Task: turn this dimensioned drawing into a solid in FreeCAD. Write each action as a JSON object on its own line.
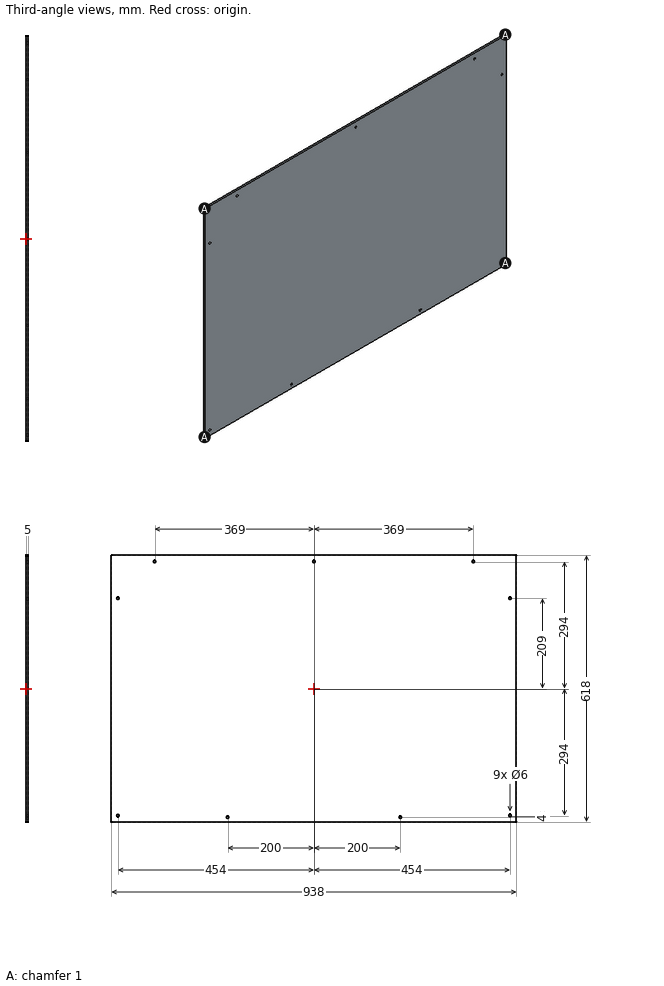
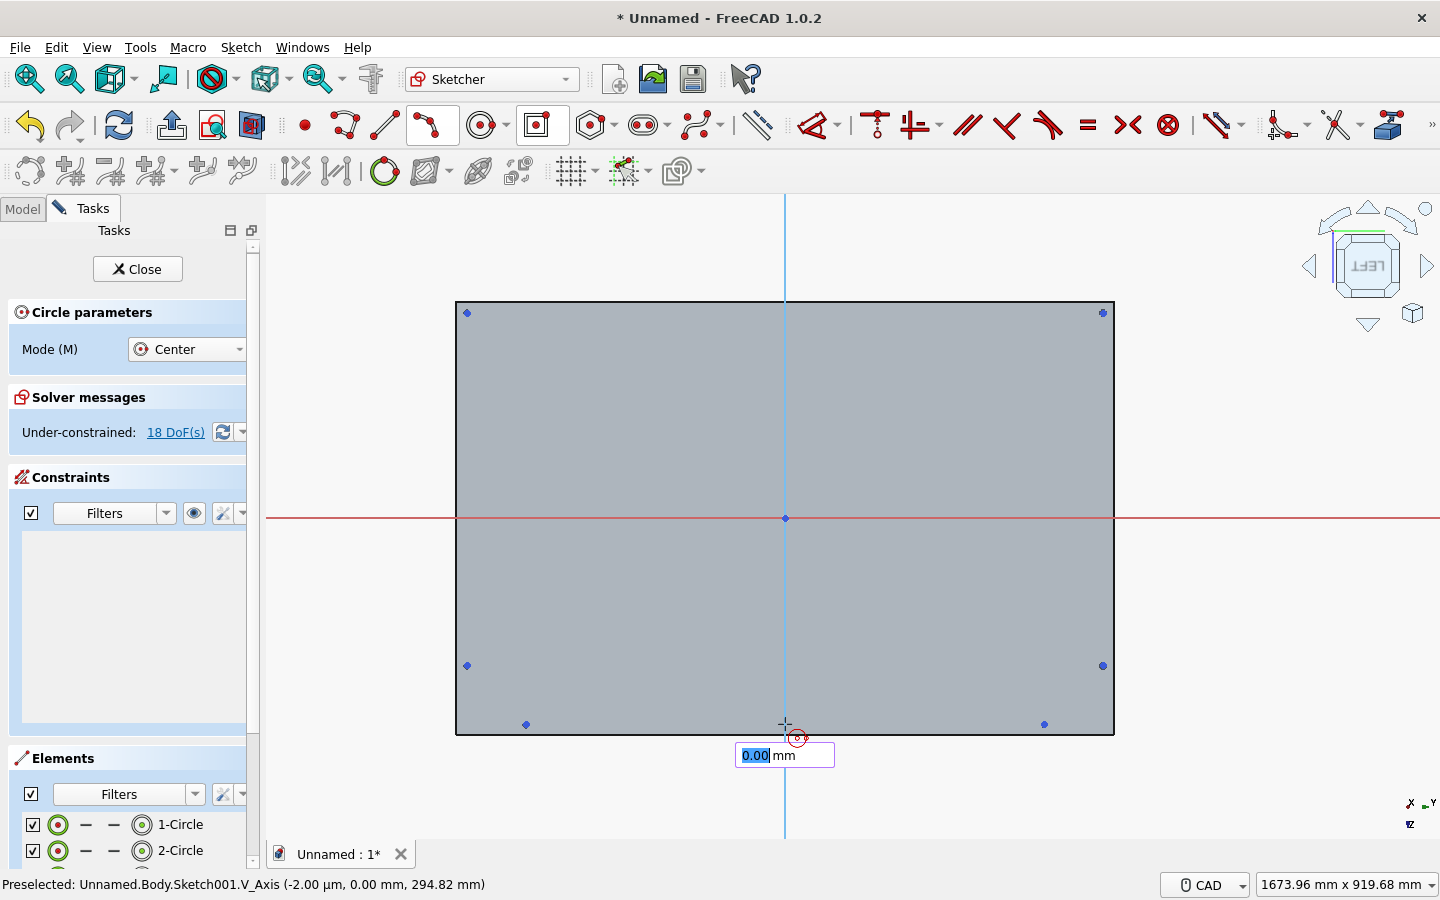
{"action": "scroll", "coordinate": [787, 724], "scroll_direction": "up", "scroll_amount": 11}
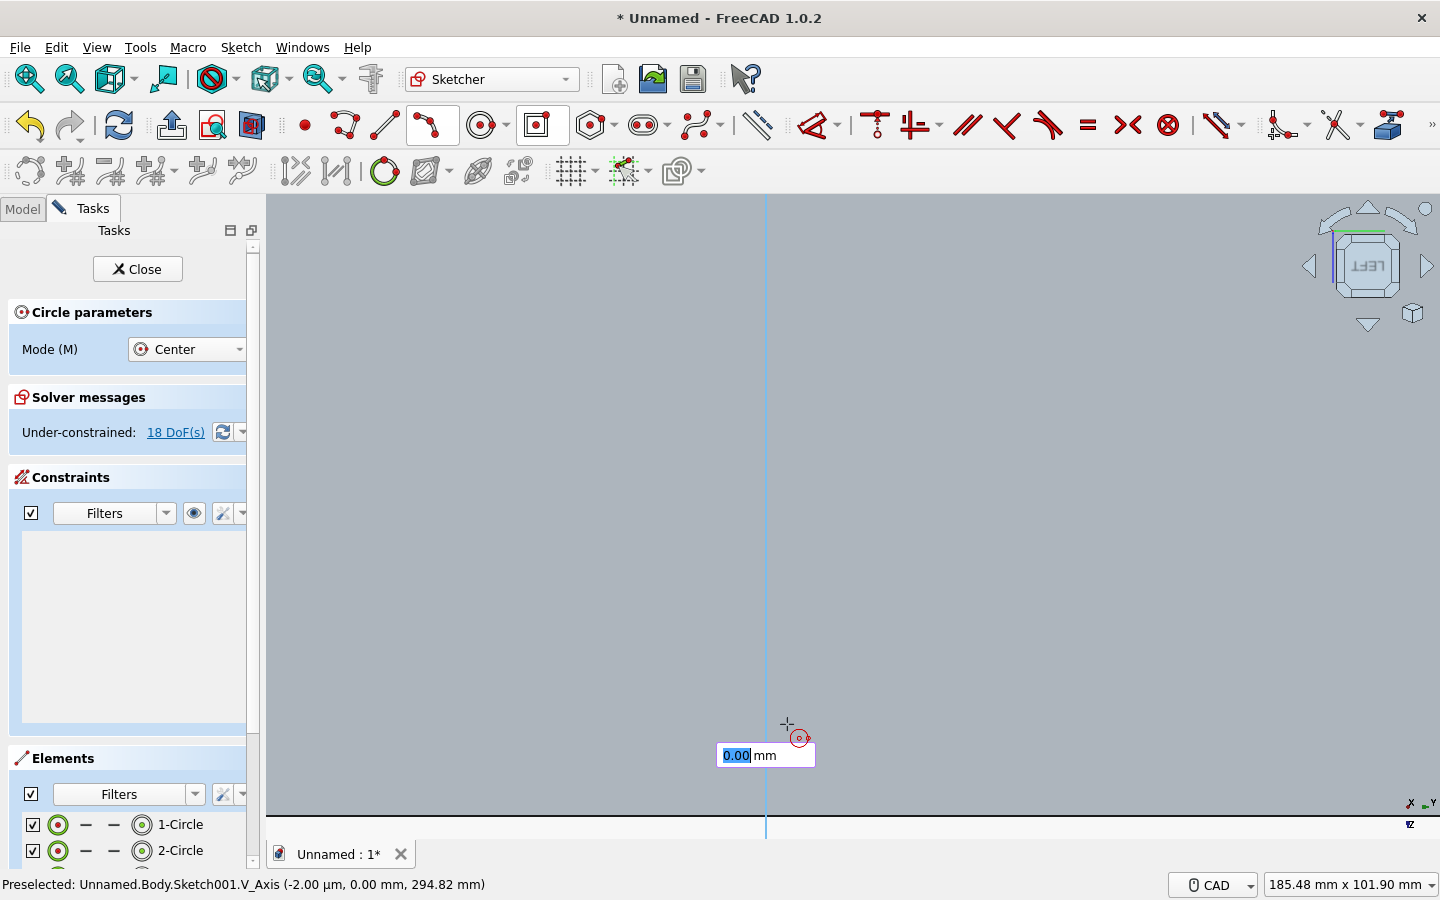
{"action": "left_click", "coordinate": [784, 715]}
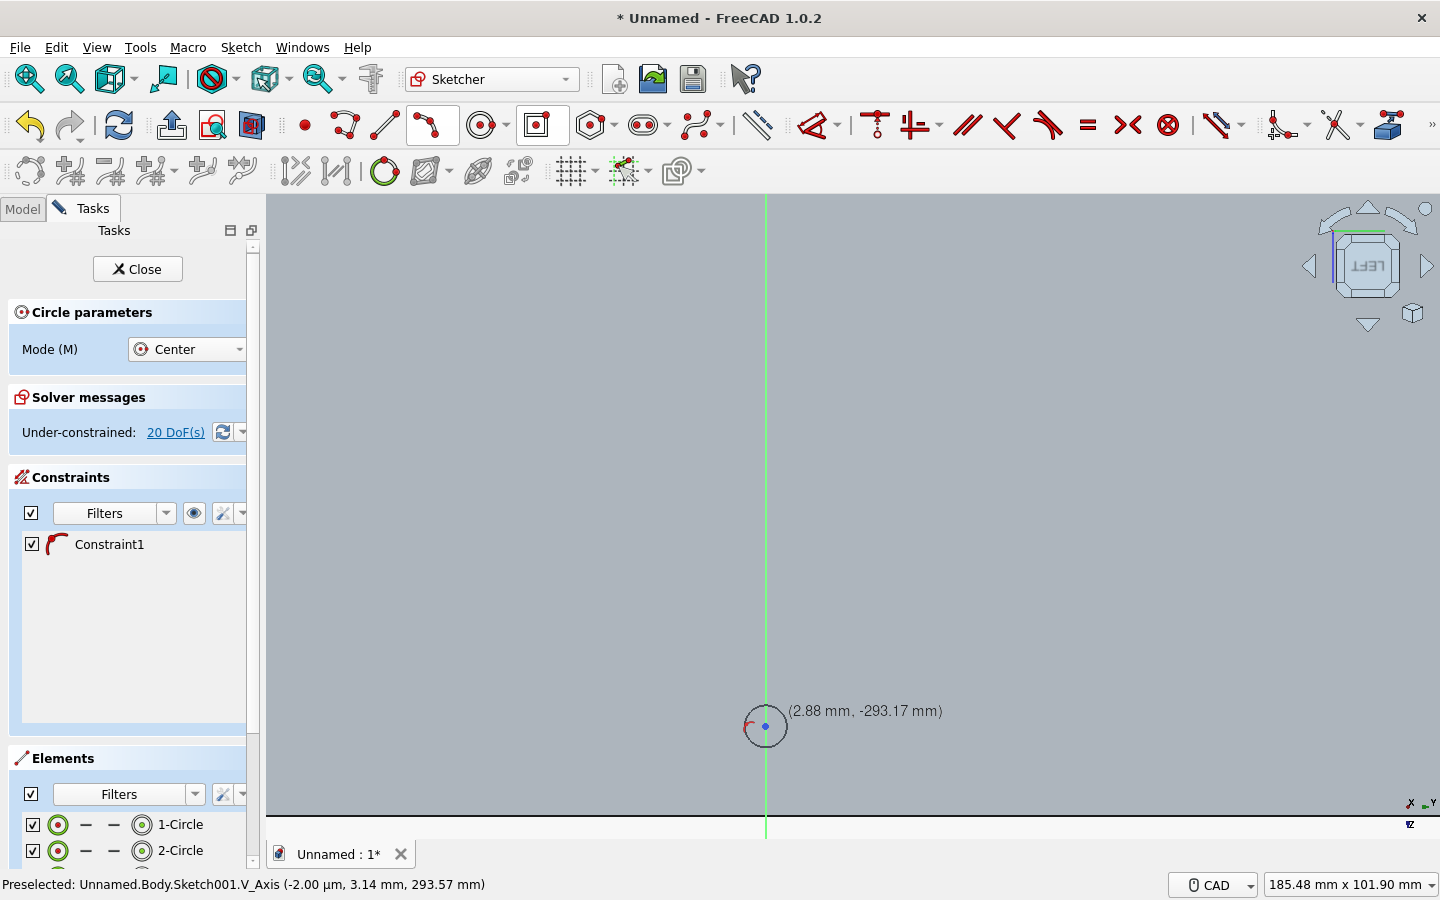
{"action": "scroll", "coordinate": [787, 724], "scroll_direction": "down", "scroll_amount": 11}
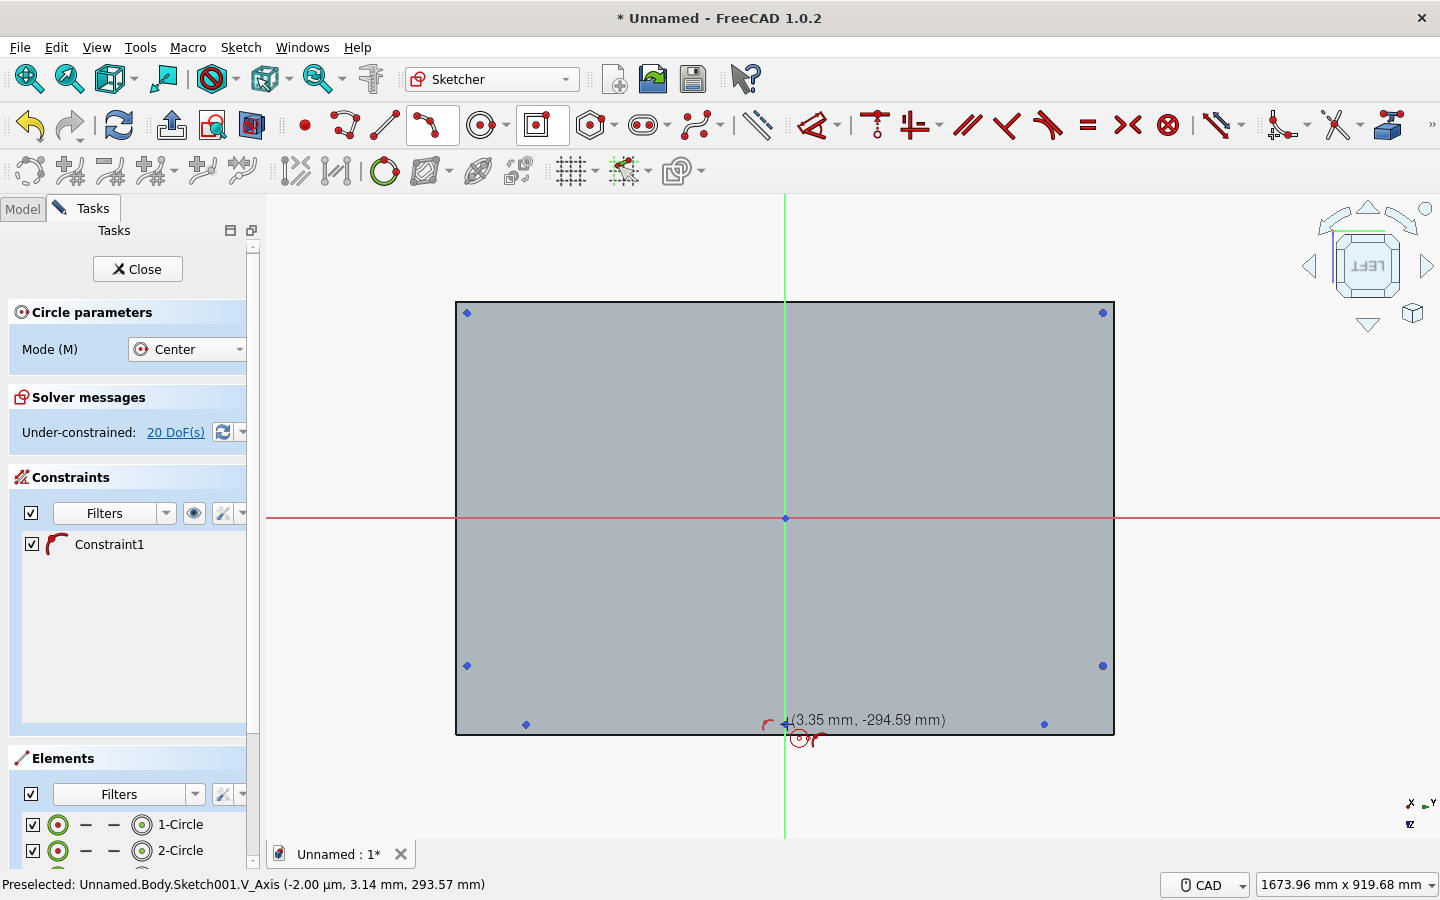
{"action": "scroll", "coordinate": [925, 309], "scroll_direction": "up", "scroll_amount": 12}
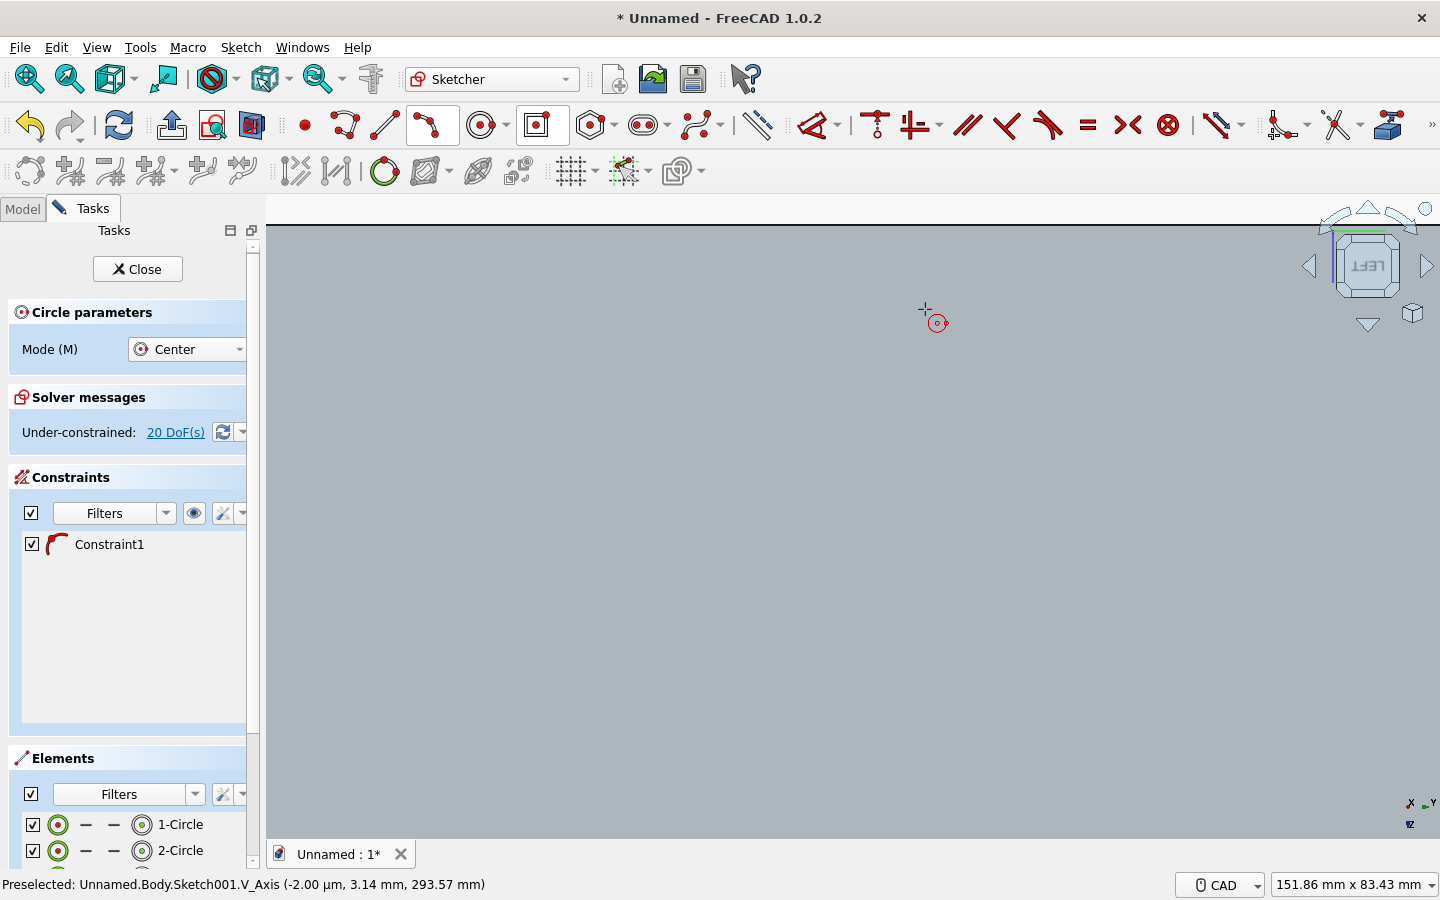
{"action": "scroll", "coordinate": [925, 309], "scroll_direction": "down", "scroll_amount": 12}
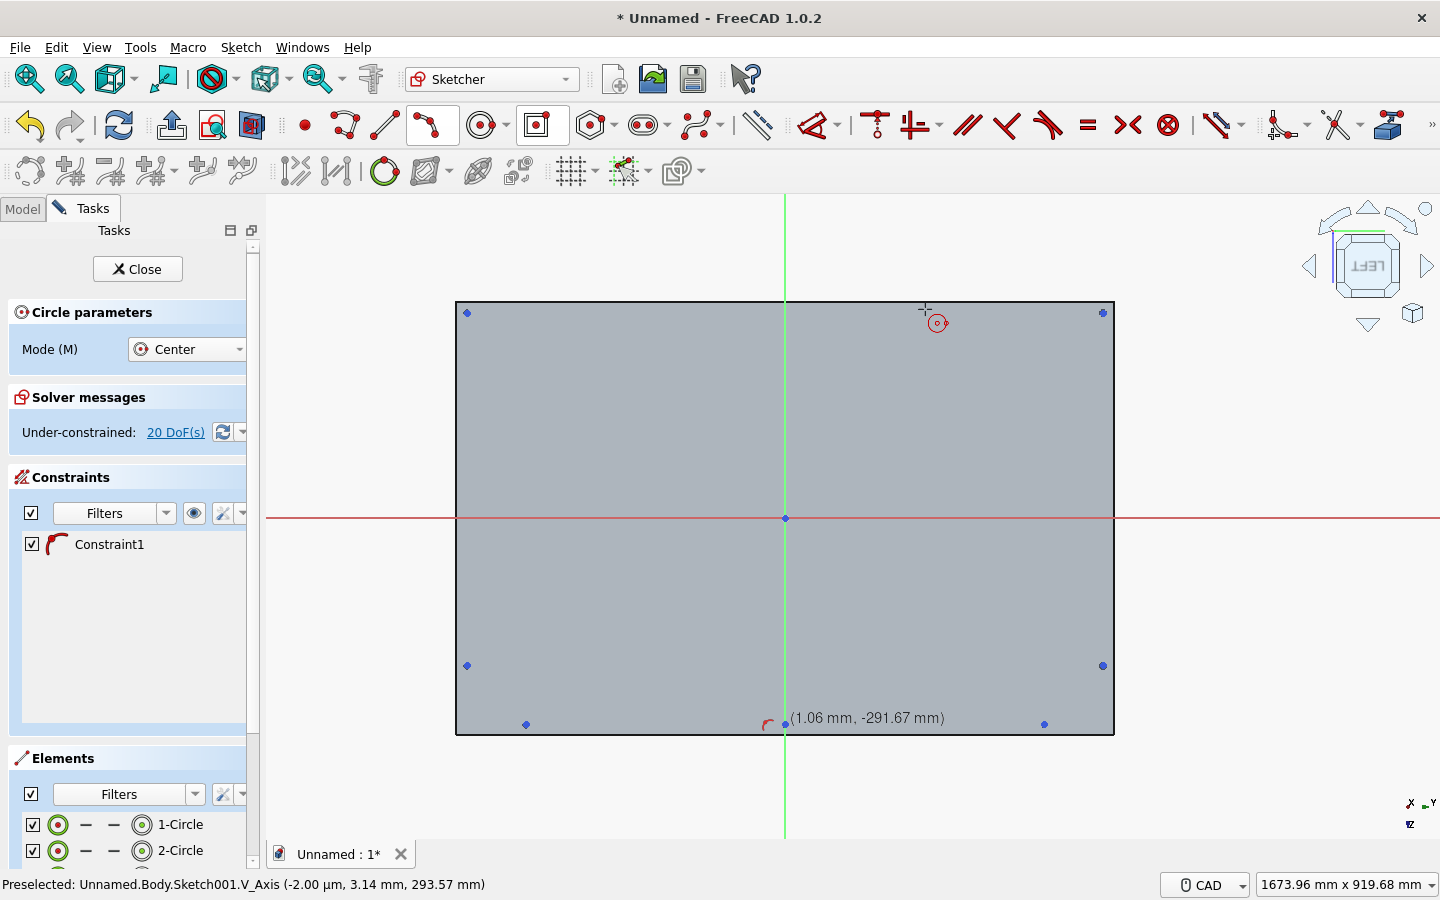
{"action": "left_click", "coordinate": [925, 309]}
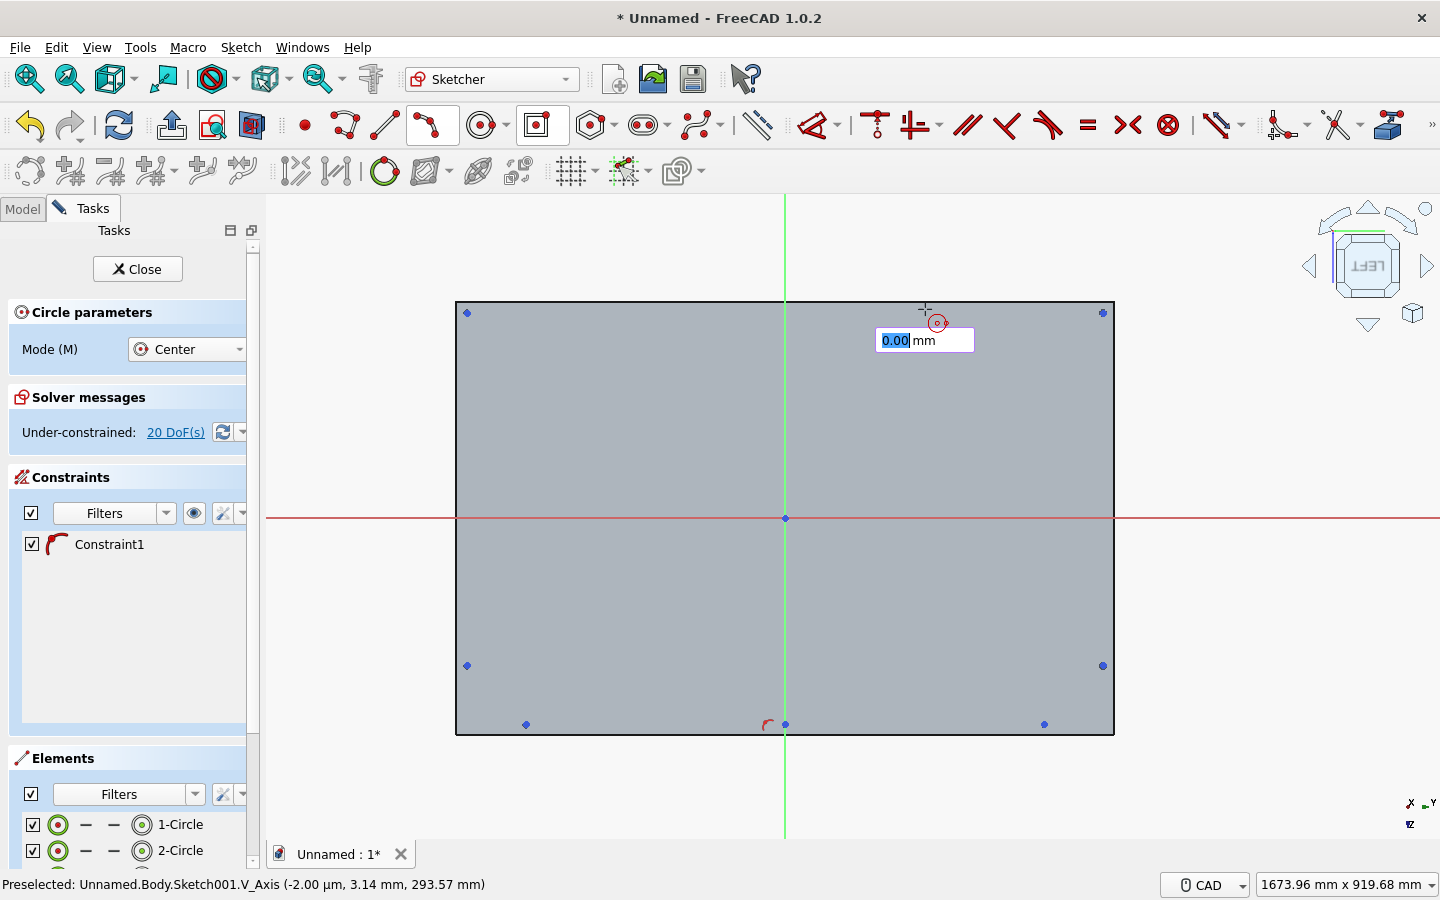
{"action": "scroll", "coordinate": [927, 308], "scroll_direction": "up", "scroll_amount": 11}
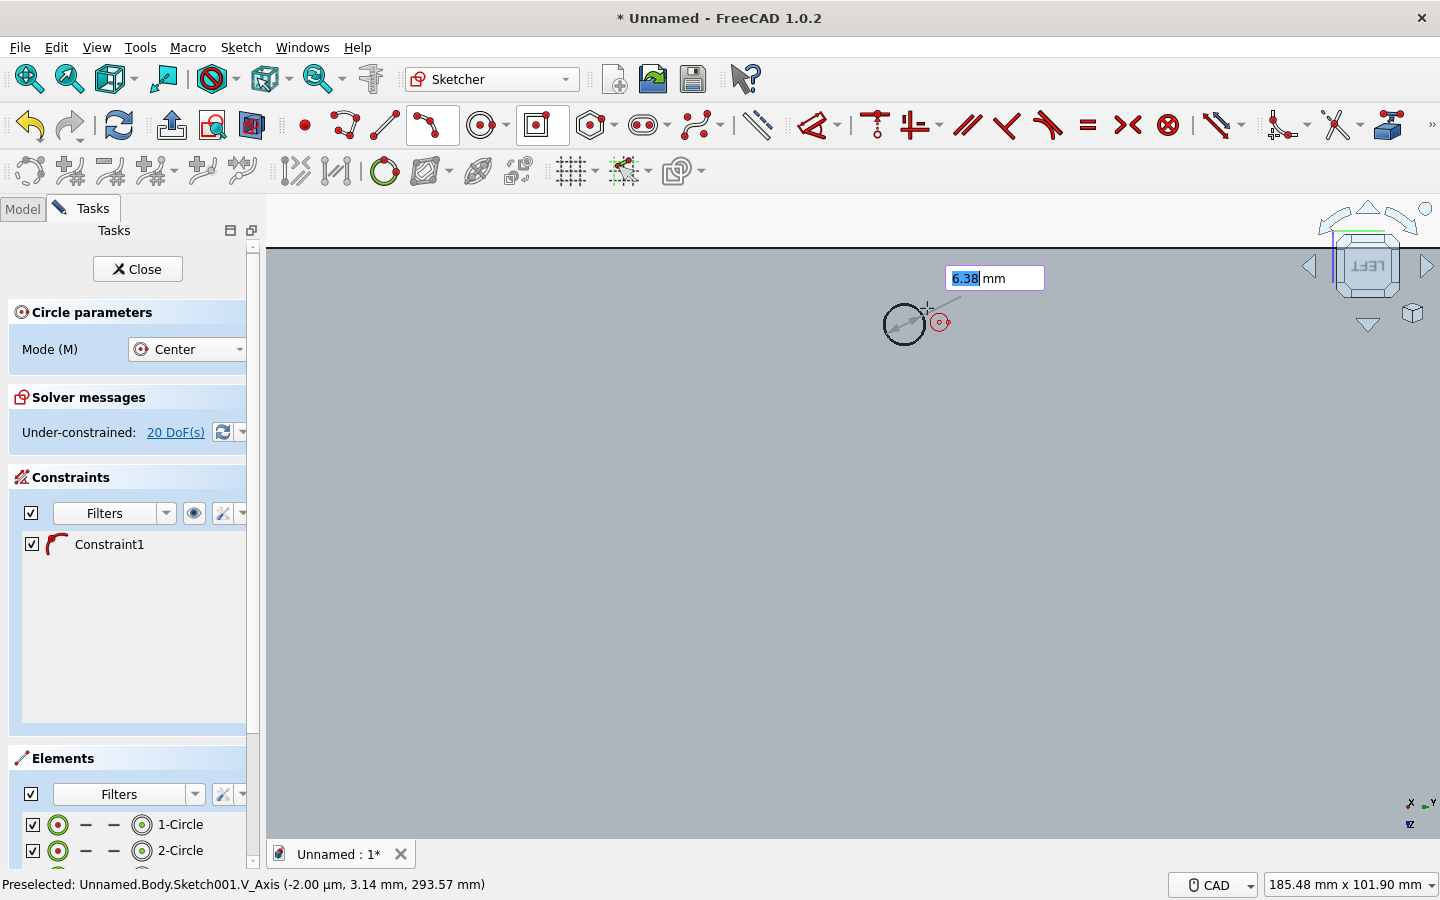
{"action": "left_click", "coordinate": [921, 304]}